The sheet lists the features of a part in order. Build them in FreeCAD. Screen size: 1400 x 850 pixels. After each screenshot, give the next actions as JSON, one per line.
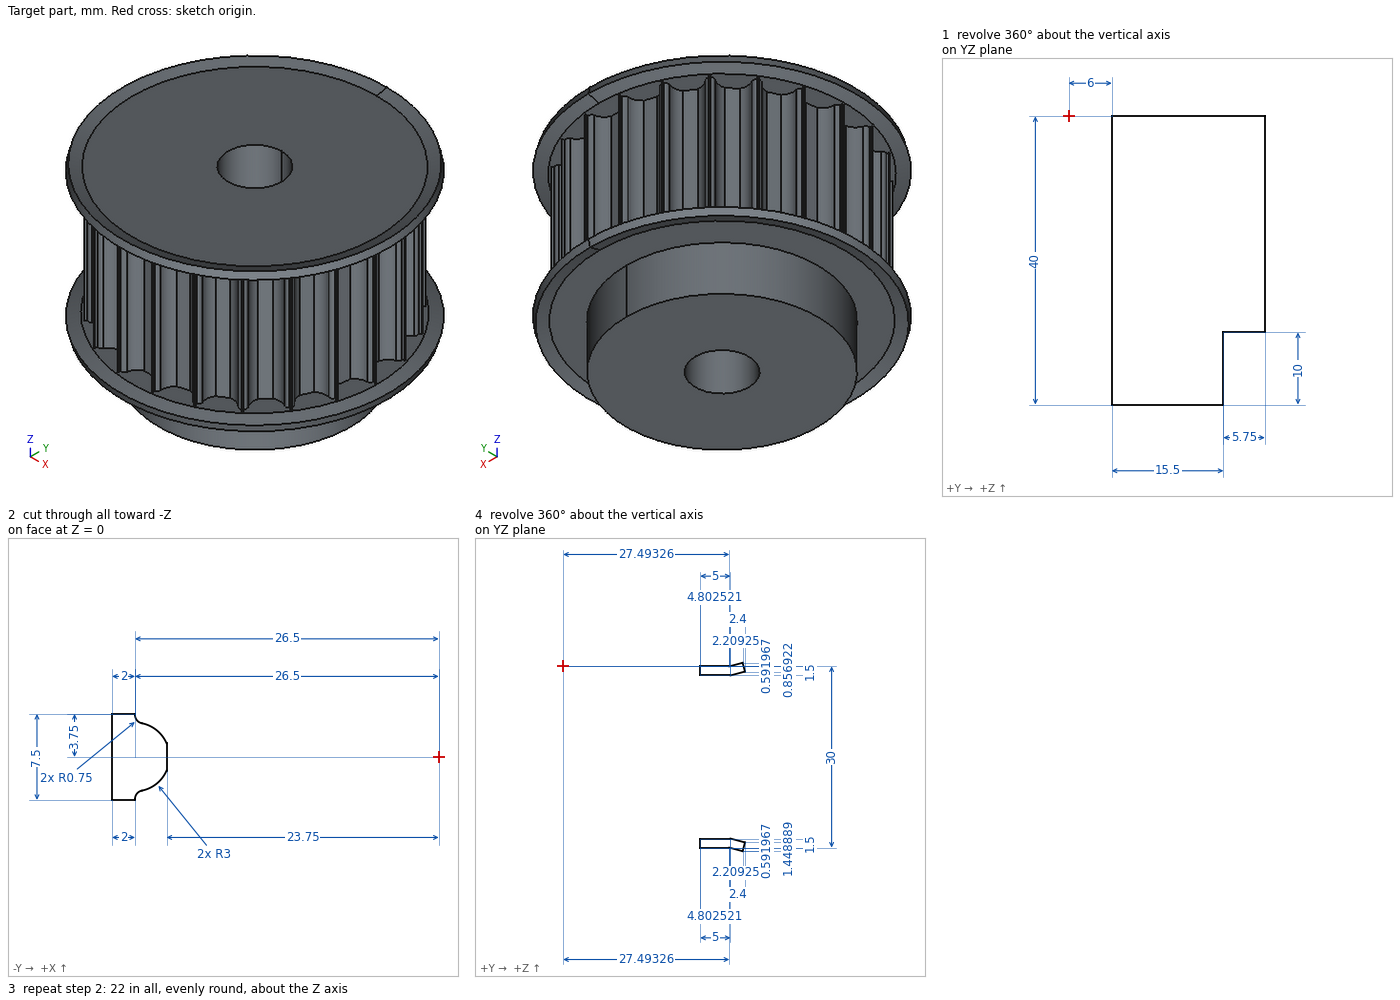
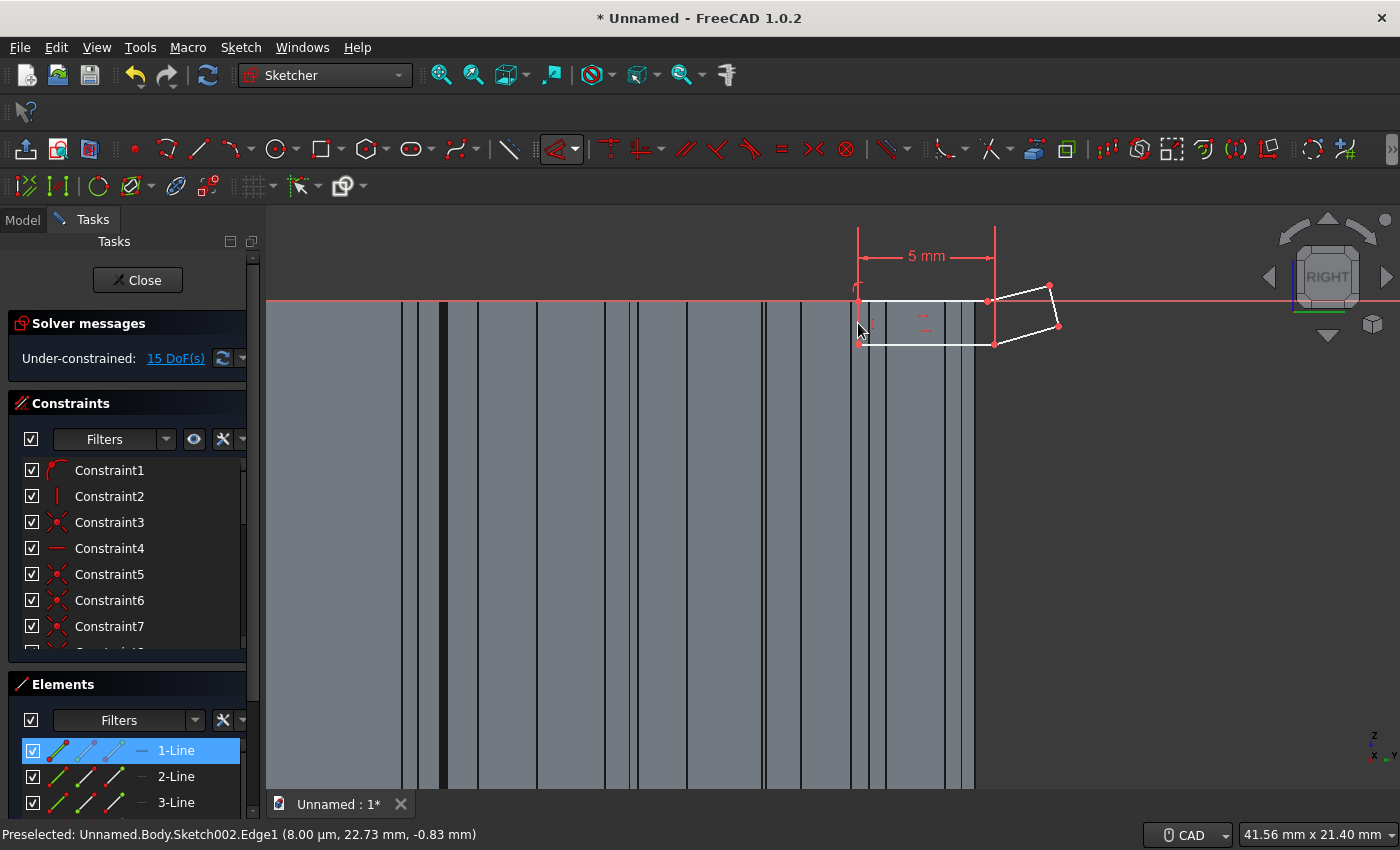
{"action": "left_click", "coordinate": [578, 150]}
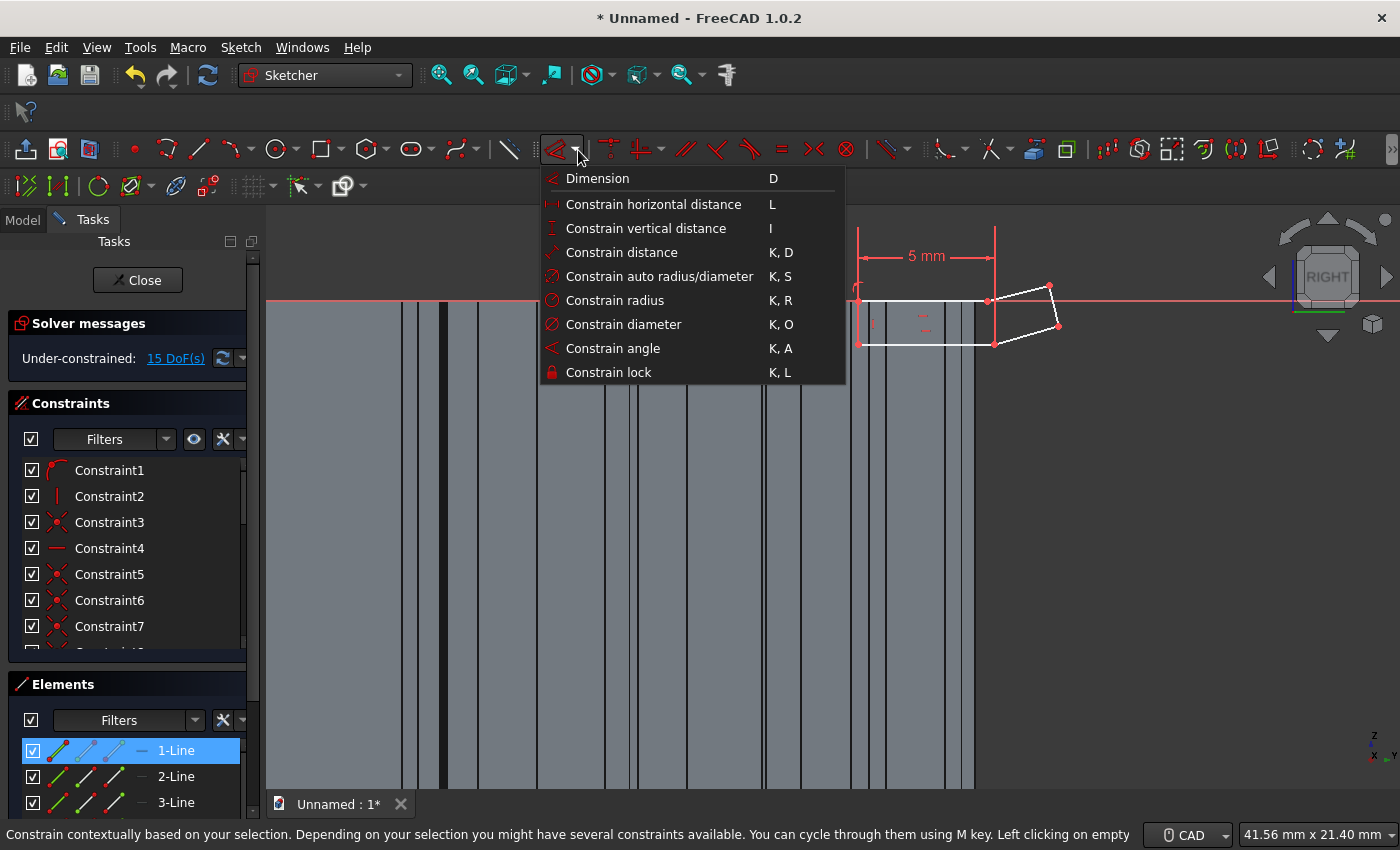
{"action": "left_click", "coordinate": [693, 228]}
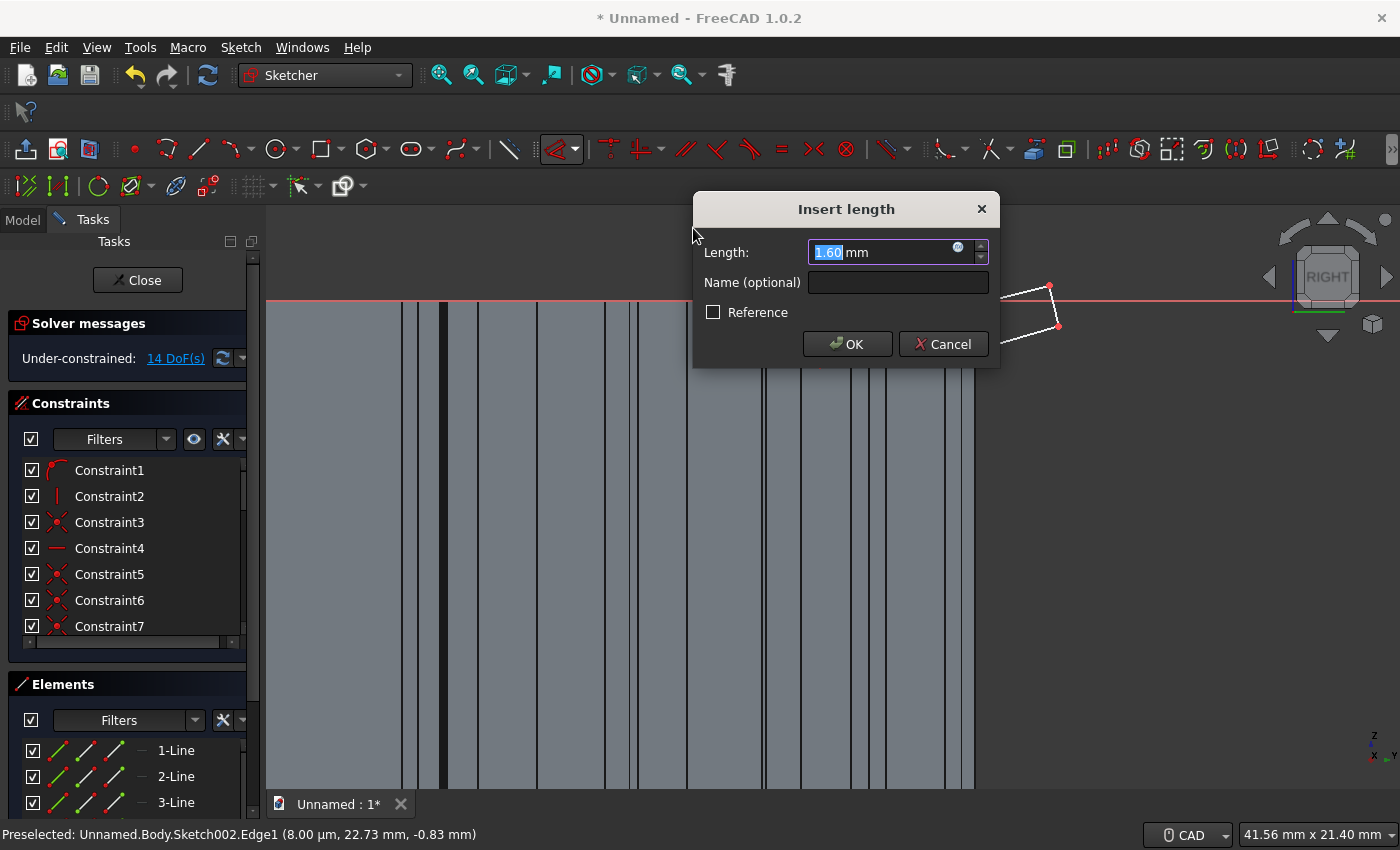
{"action": "type", "text": "1.5"}
{"action": "key", "text": "Return"}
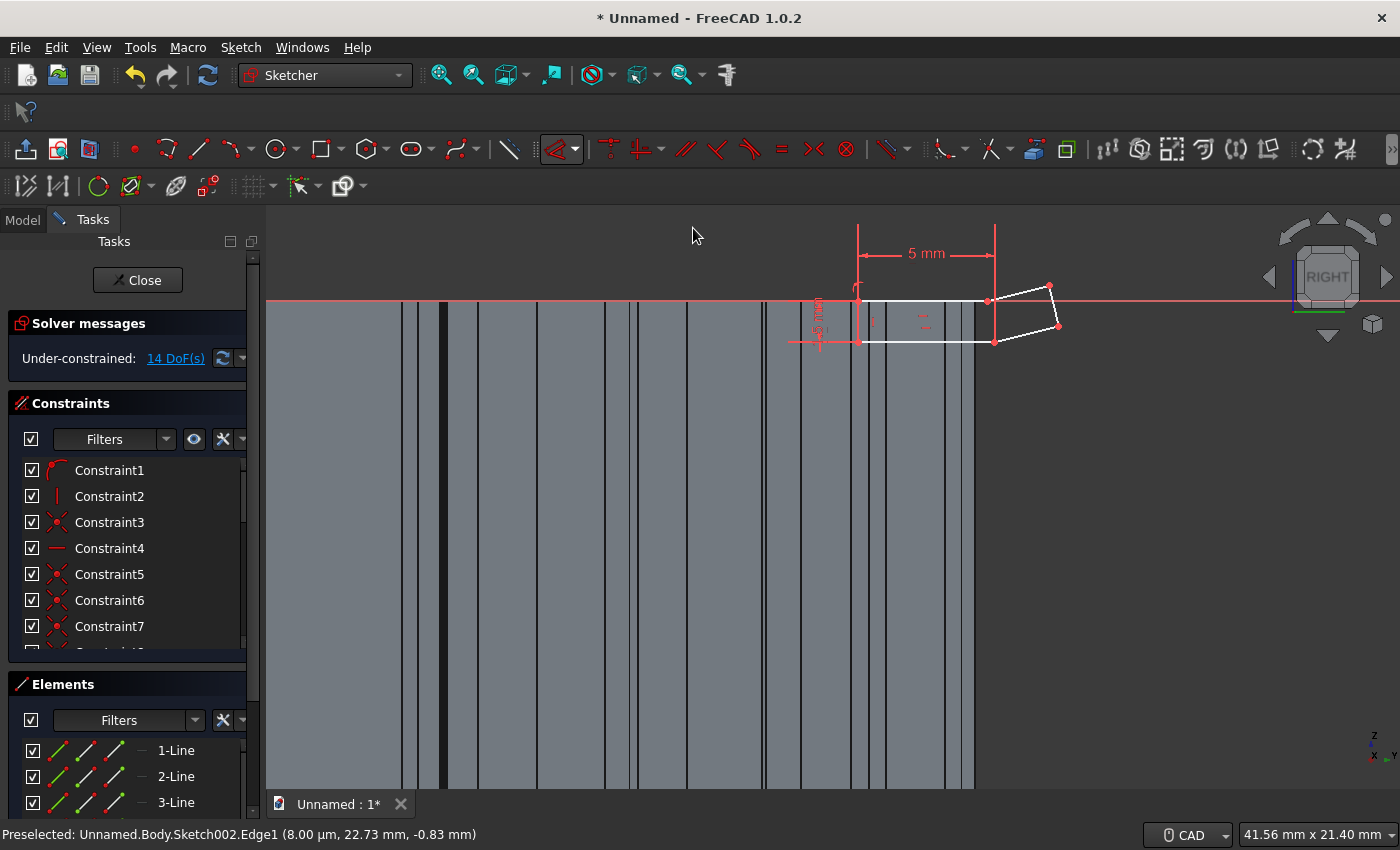
{"action": "scroll", "coordinate": [859, 323], "scroll_direction": "down", "scroll_amount": 4}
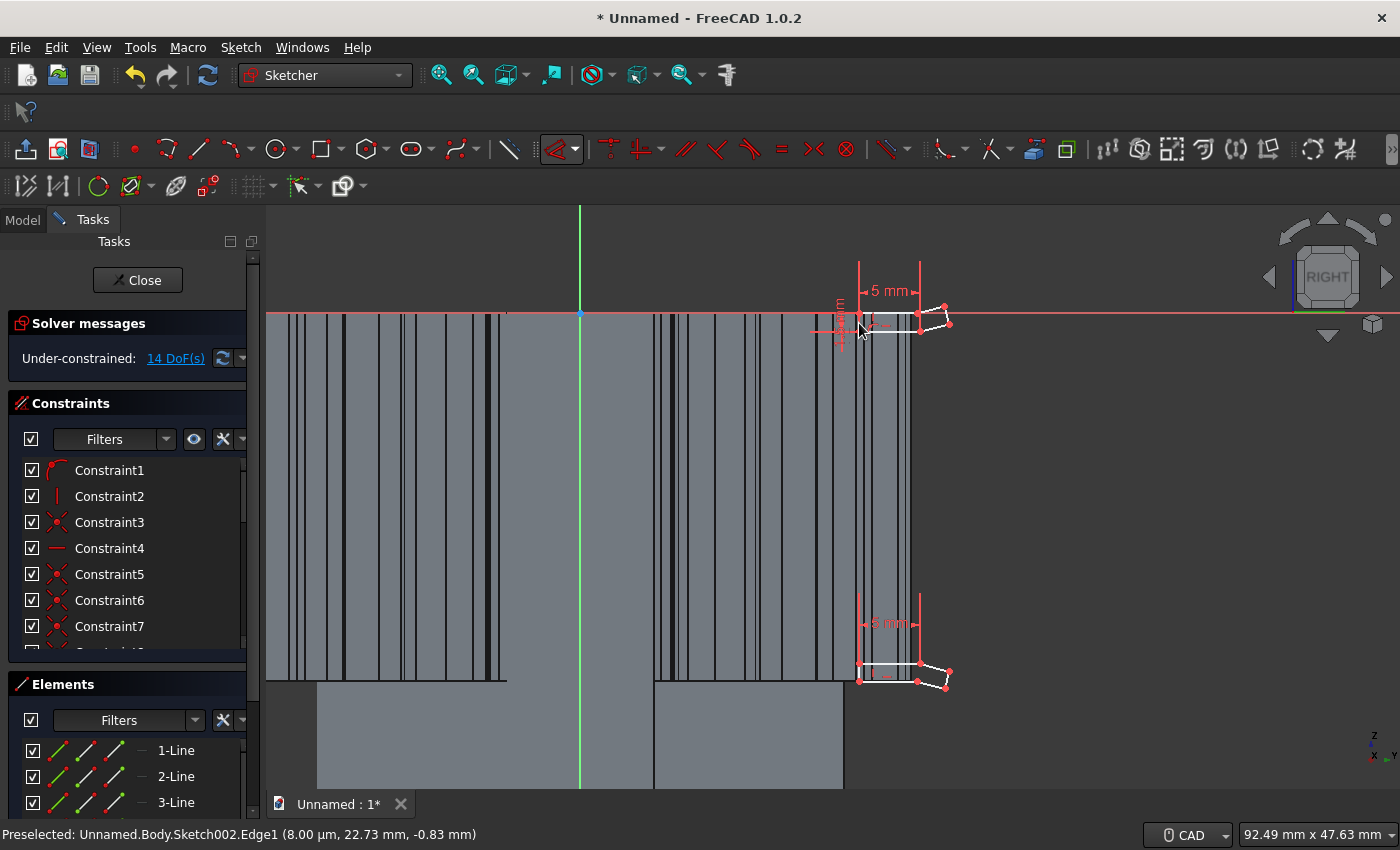
{"action": "scroll", "coordinate": [859, 669], "scroll_direction": "up", "scroll_amount": 5}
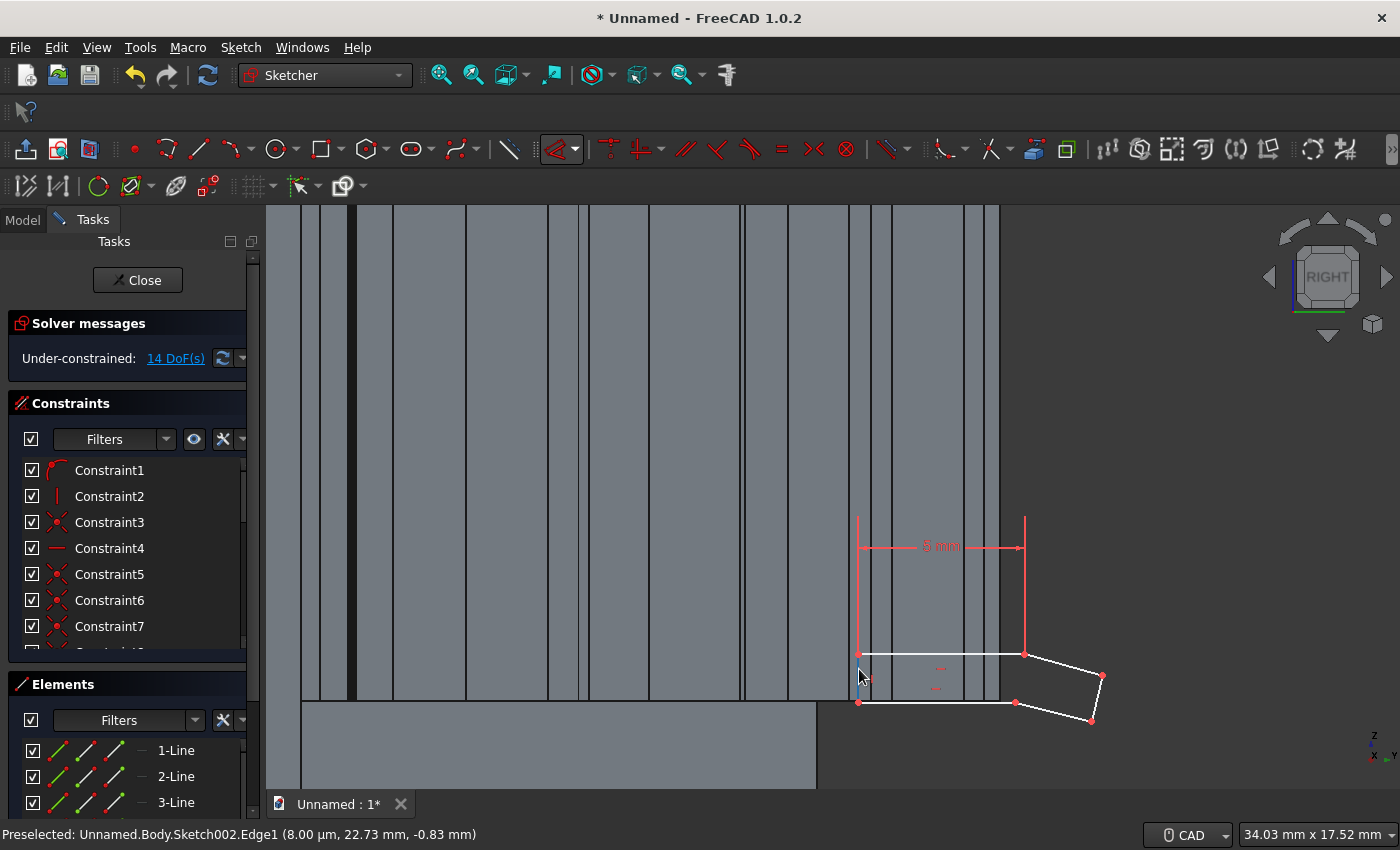
{"action": "left_click", "coordinate": [858, 669]}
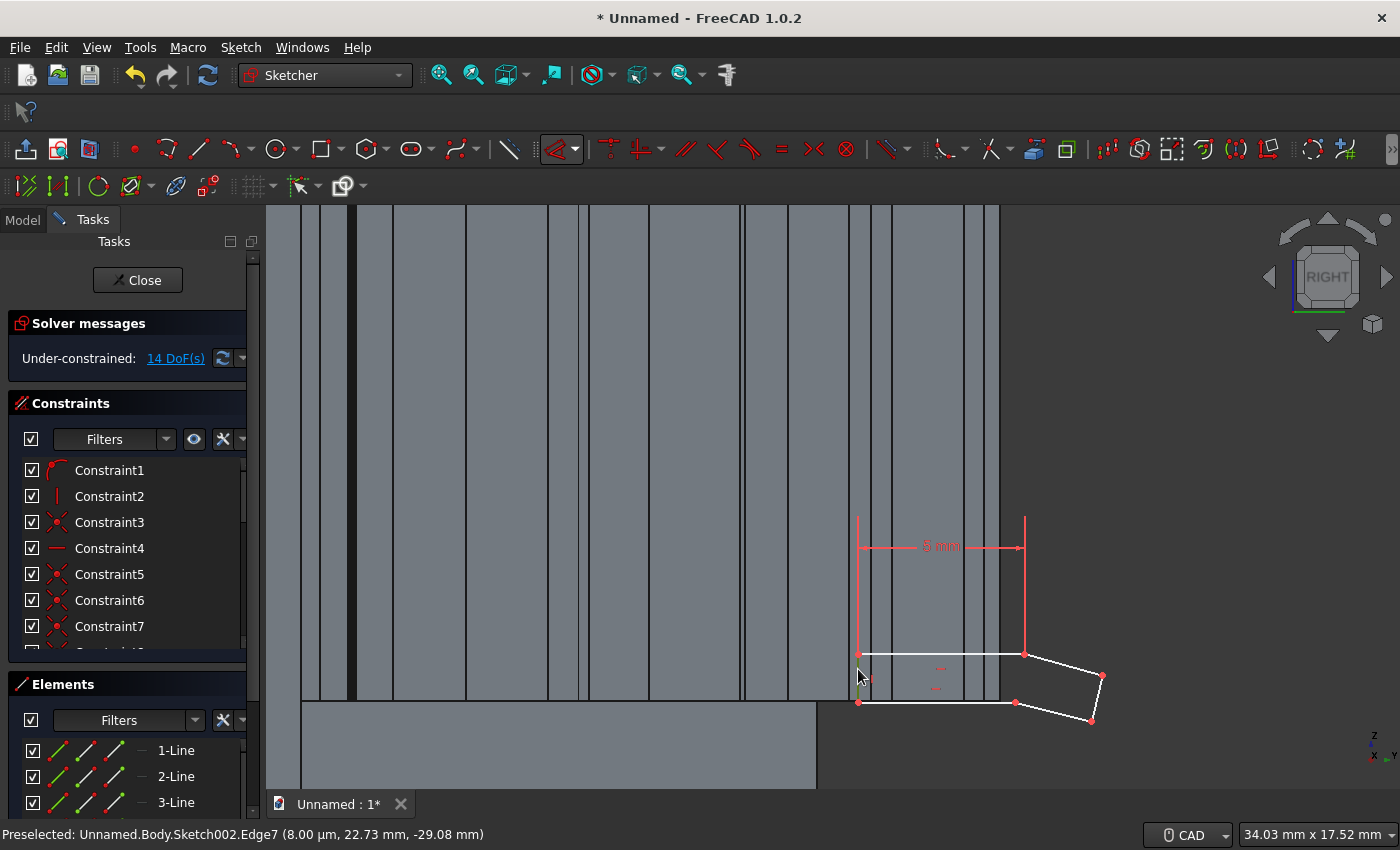
{"action": "left_click", "coordinate": [578, 150]}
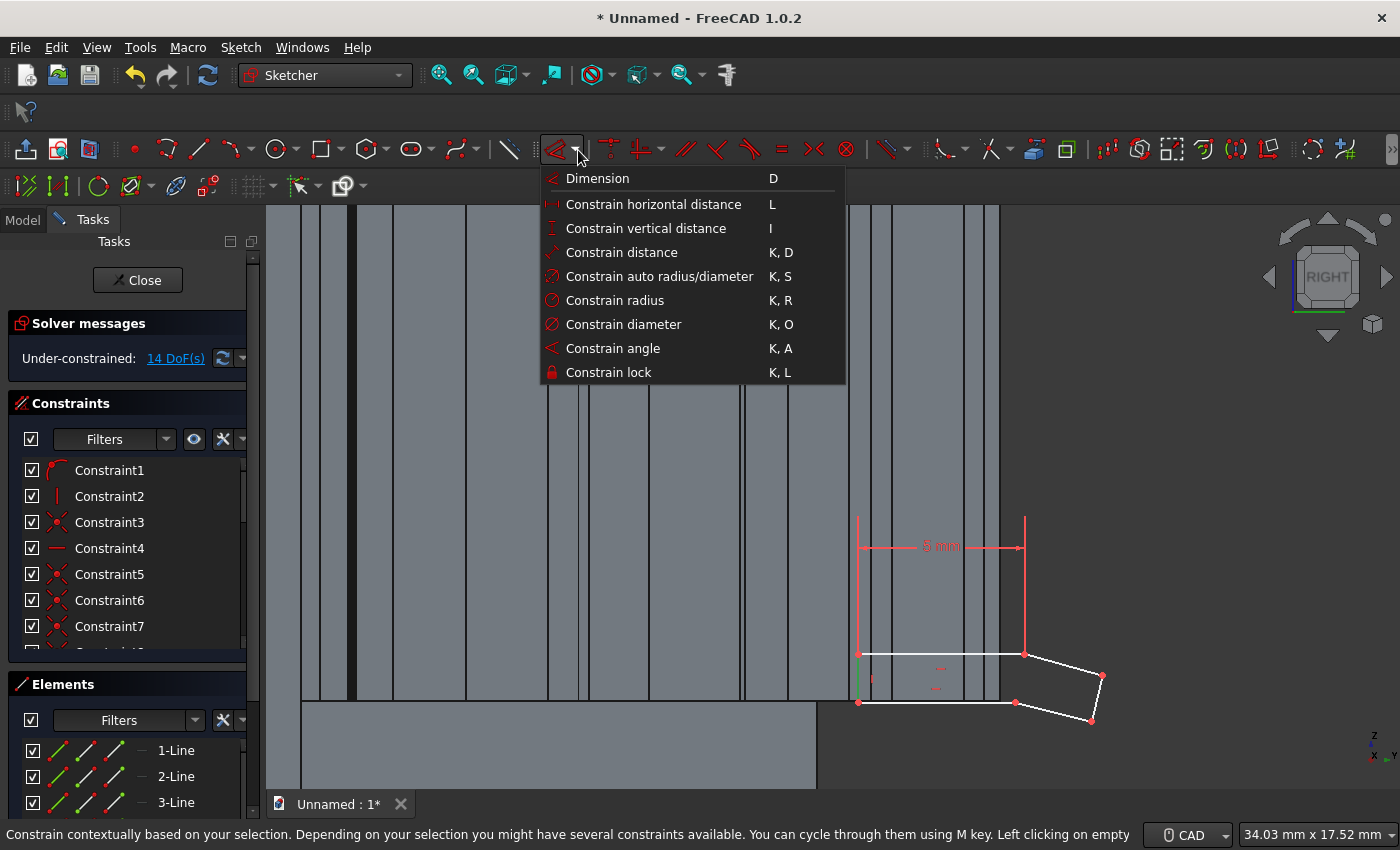
{"action": "left_click", "coordinate": [693, 228]}